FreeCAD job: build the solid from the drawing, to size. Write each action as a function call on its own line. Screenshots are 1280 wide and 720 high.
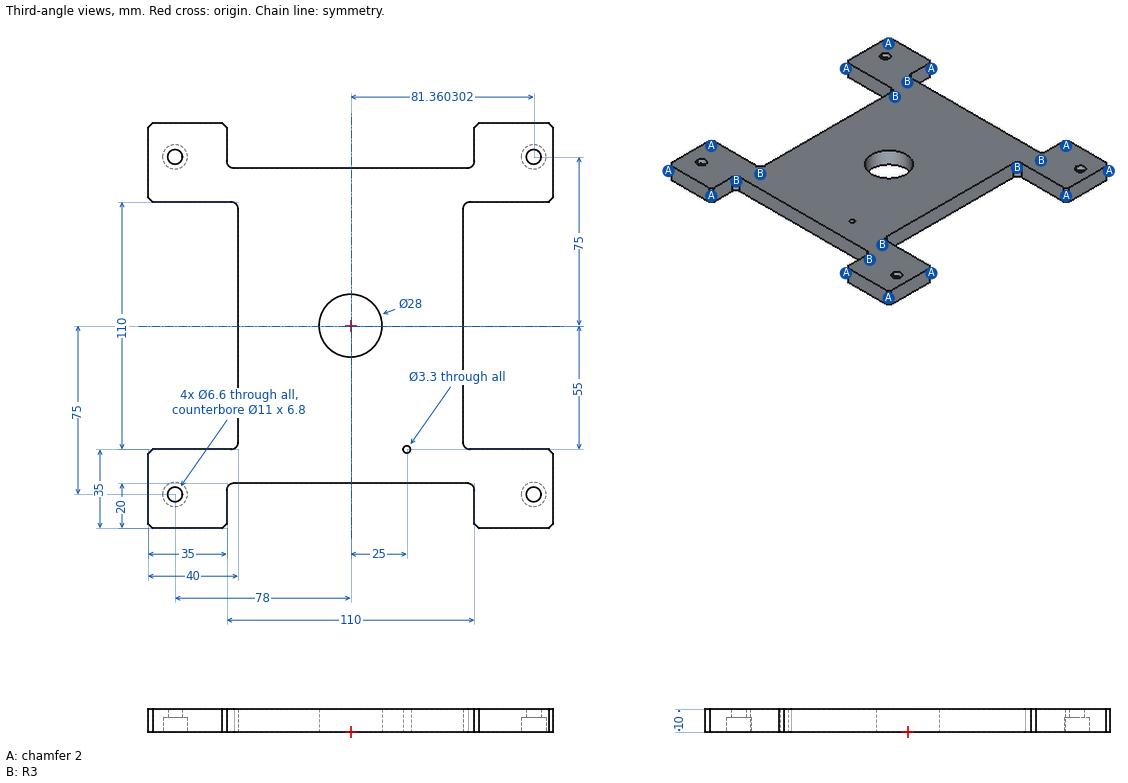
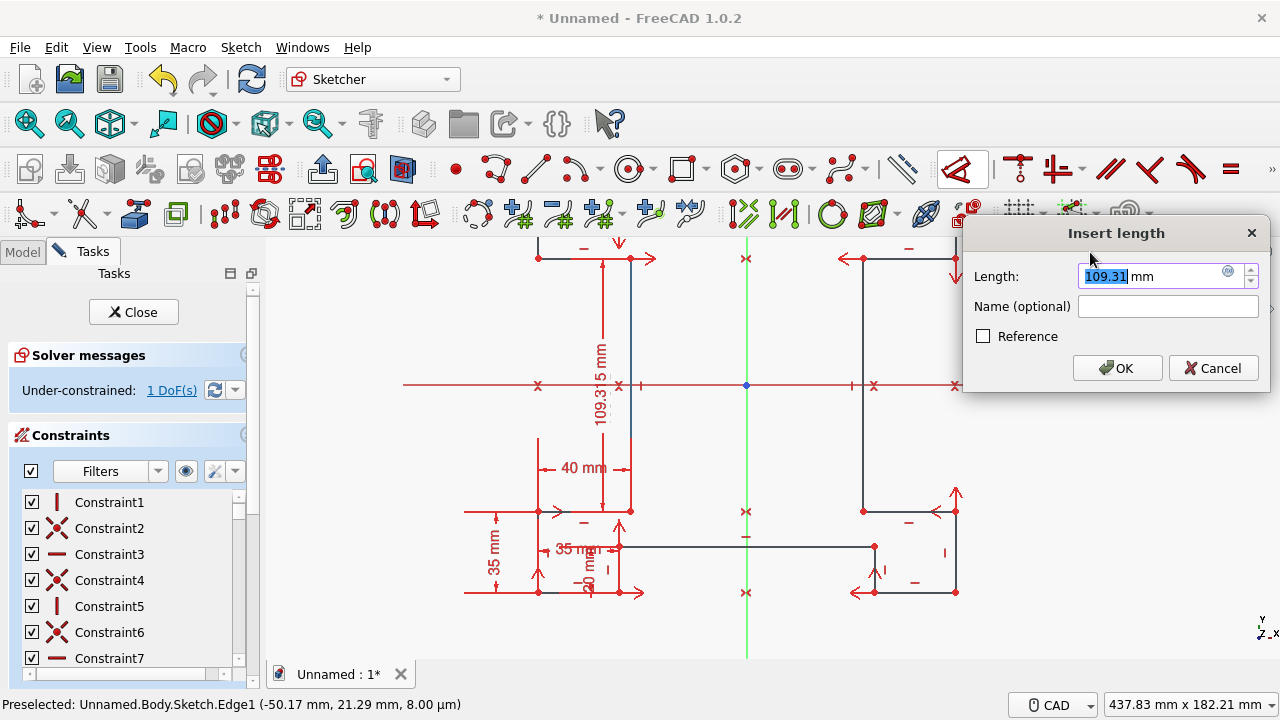
text(110)
key(Return)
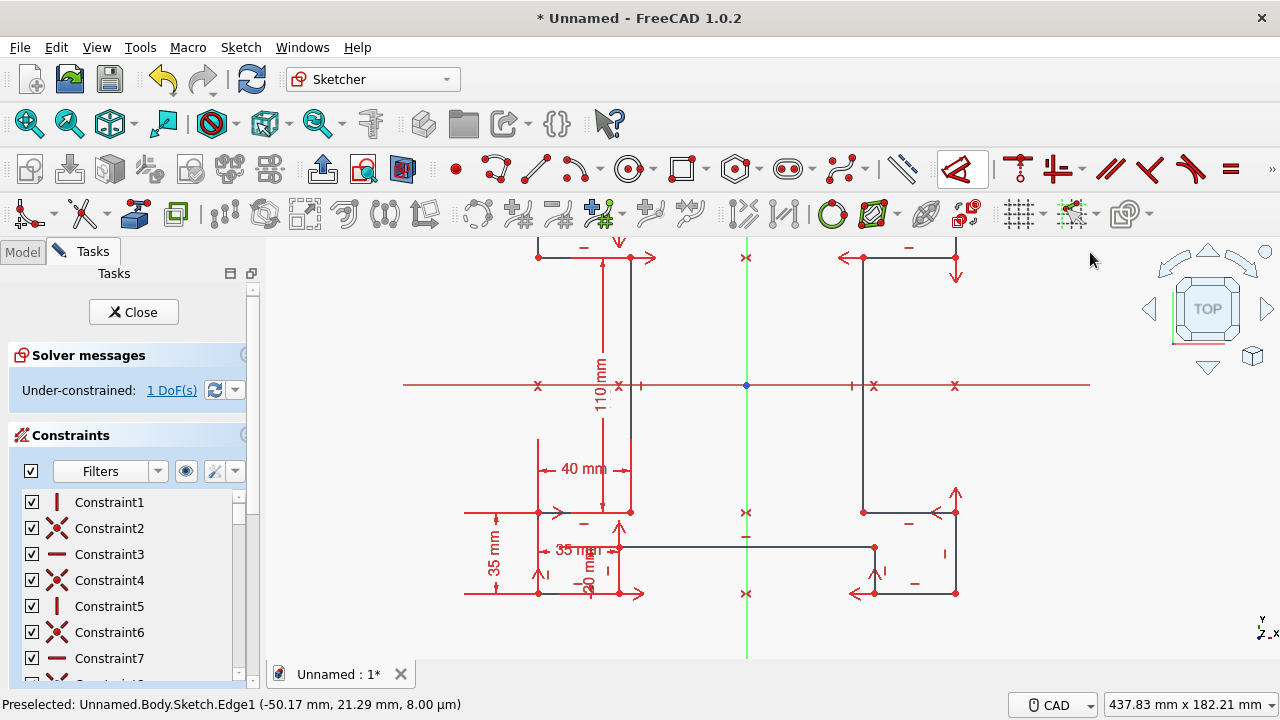
click(696, 547)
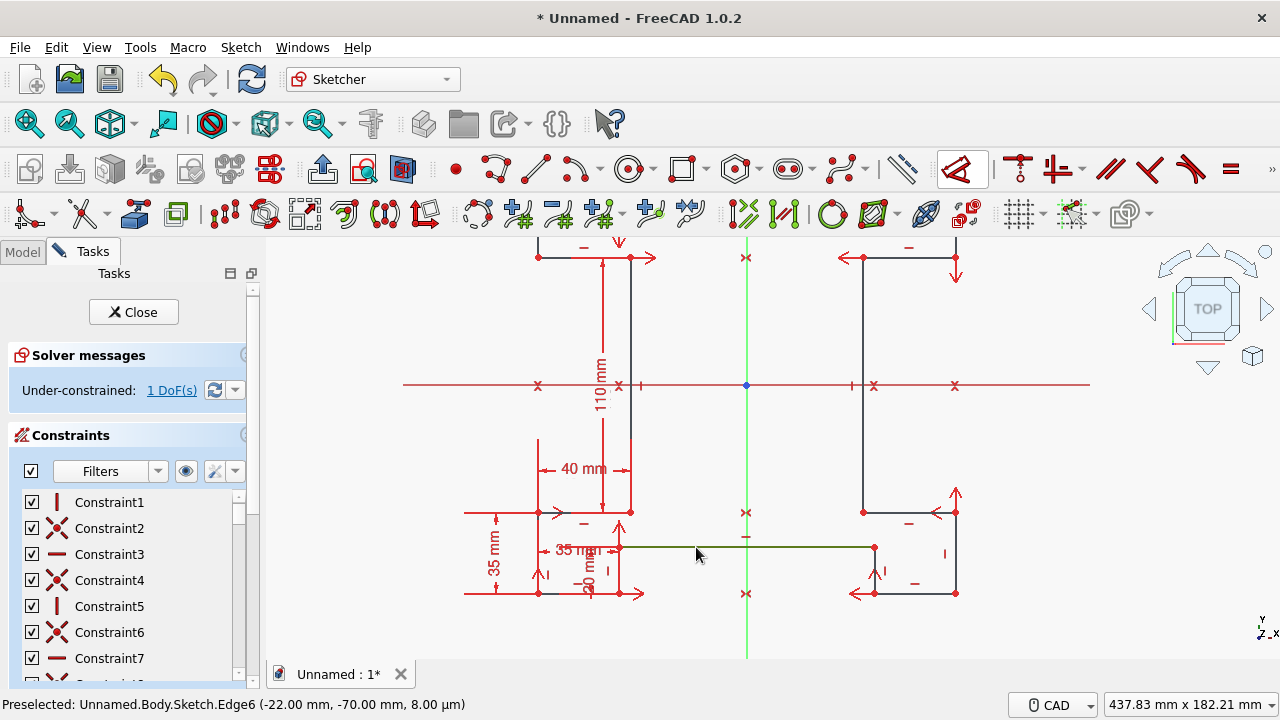
key(l)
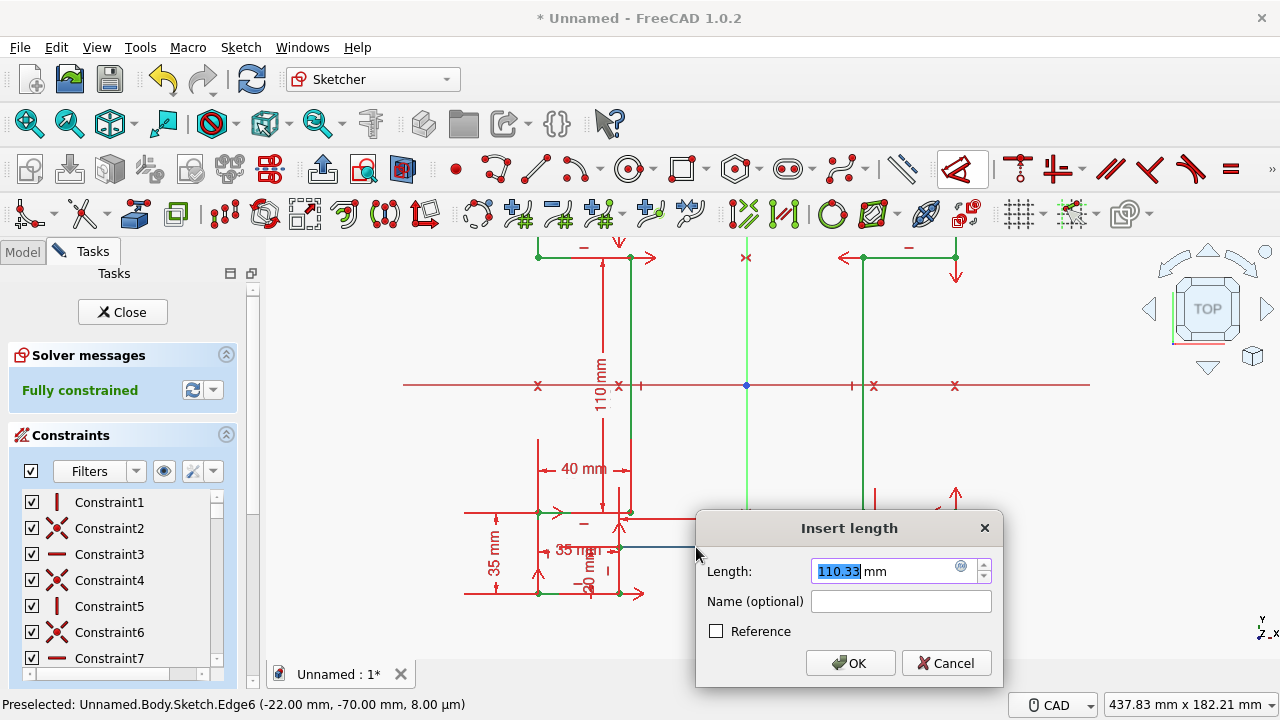
text(110)
key(Return)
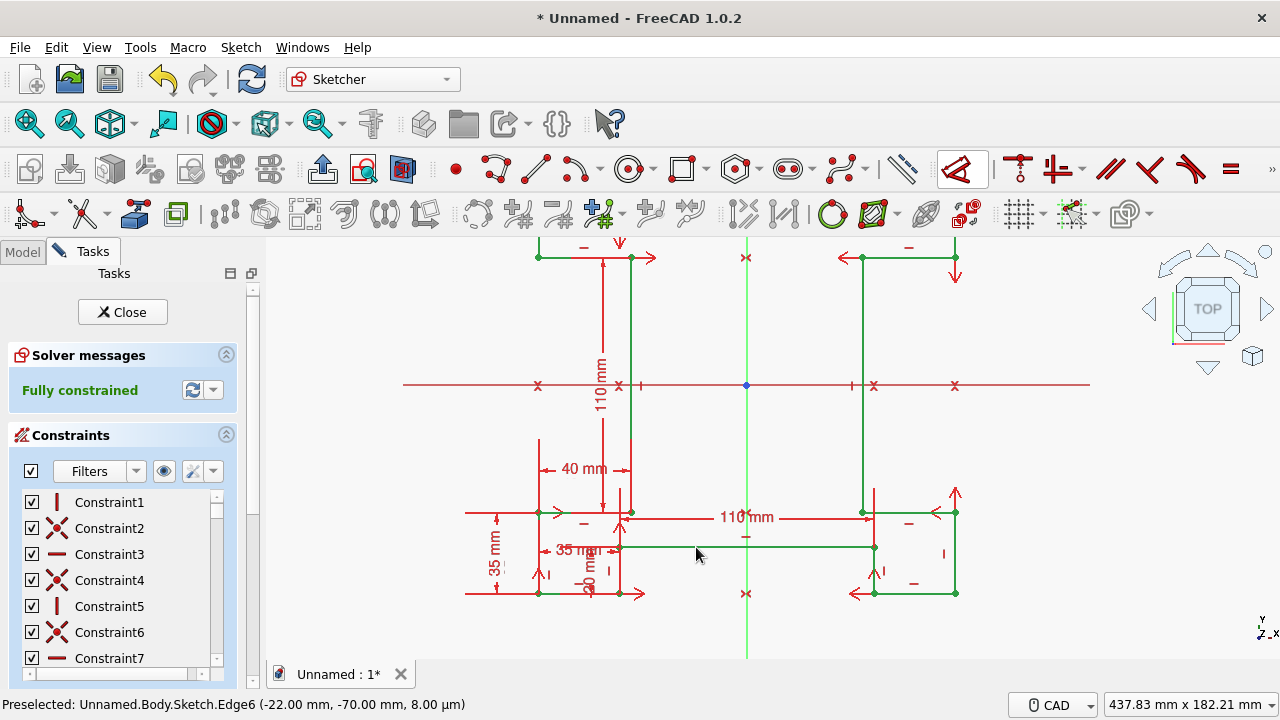
click(123, 312)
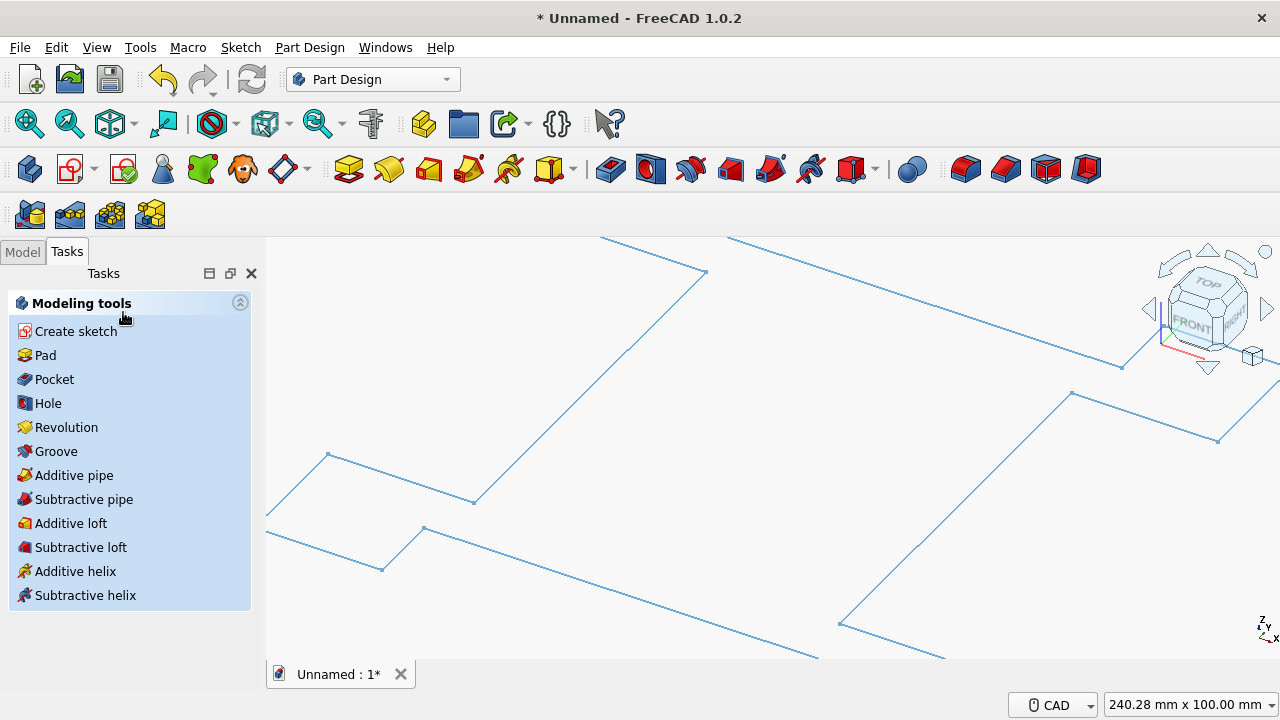
click(350, 170)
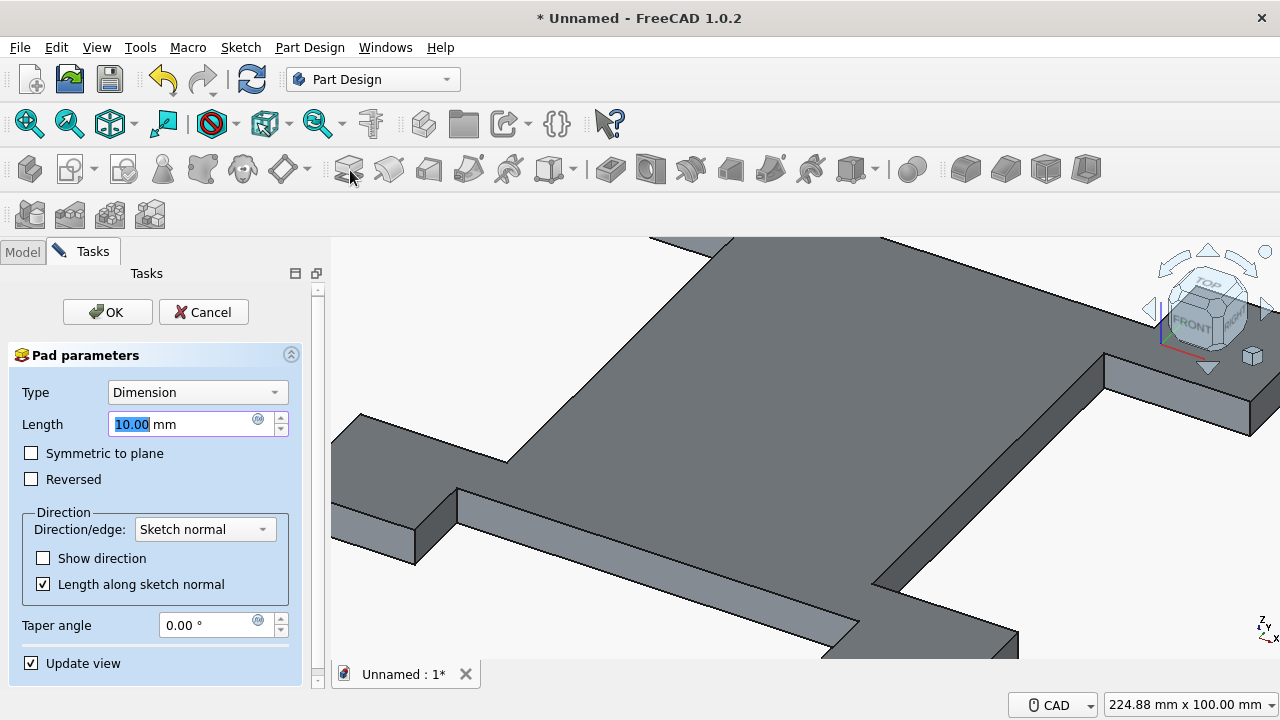
text(10)
key(Tab)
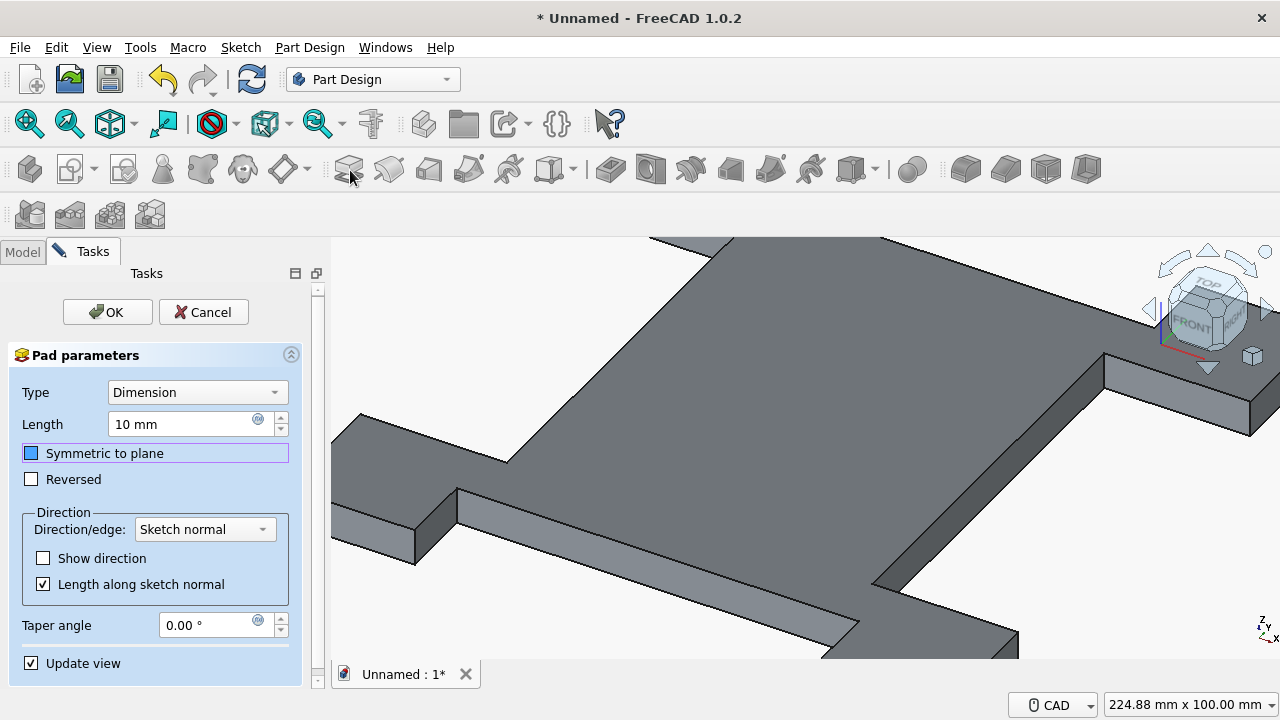
click(108, 312)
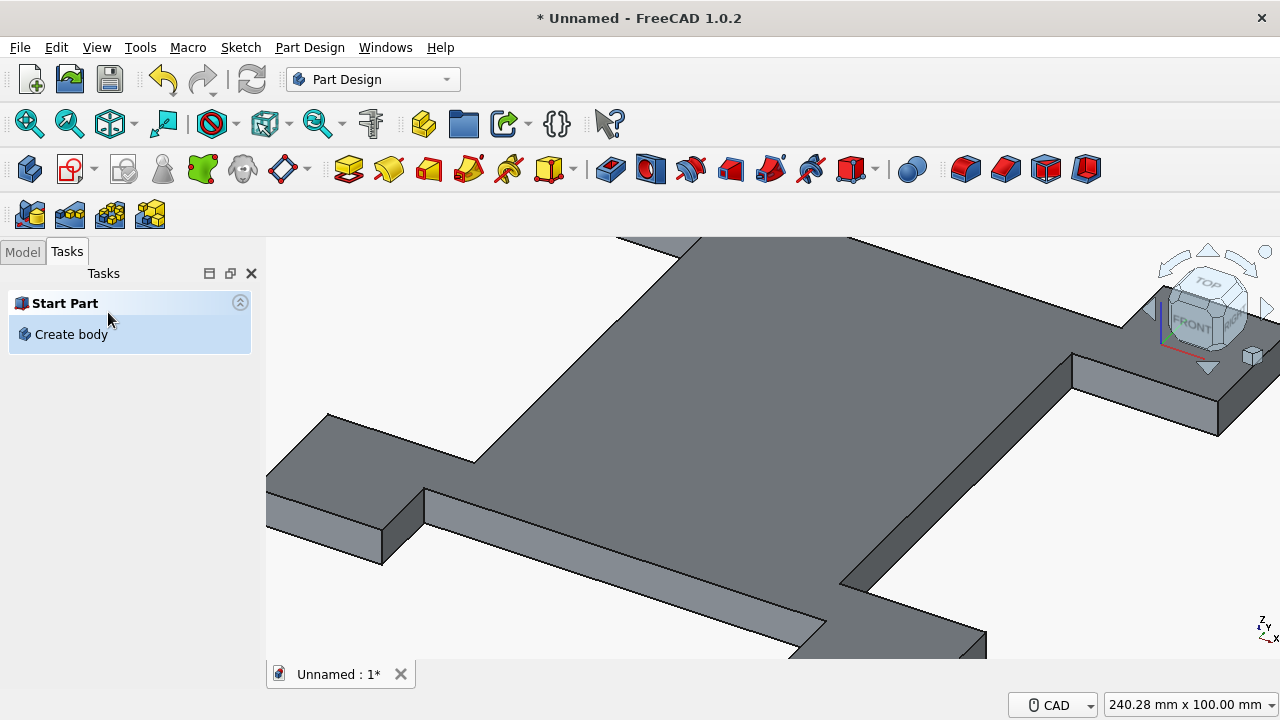
click(30, 124)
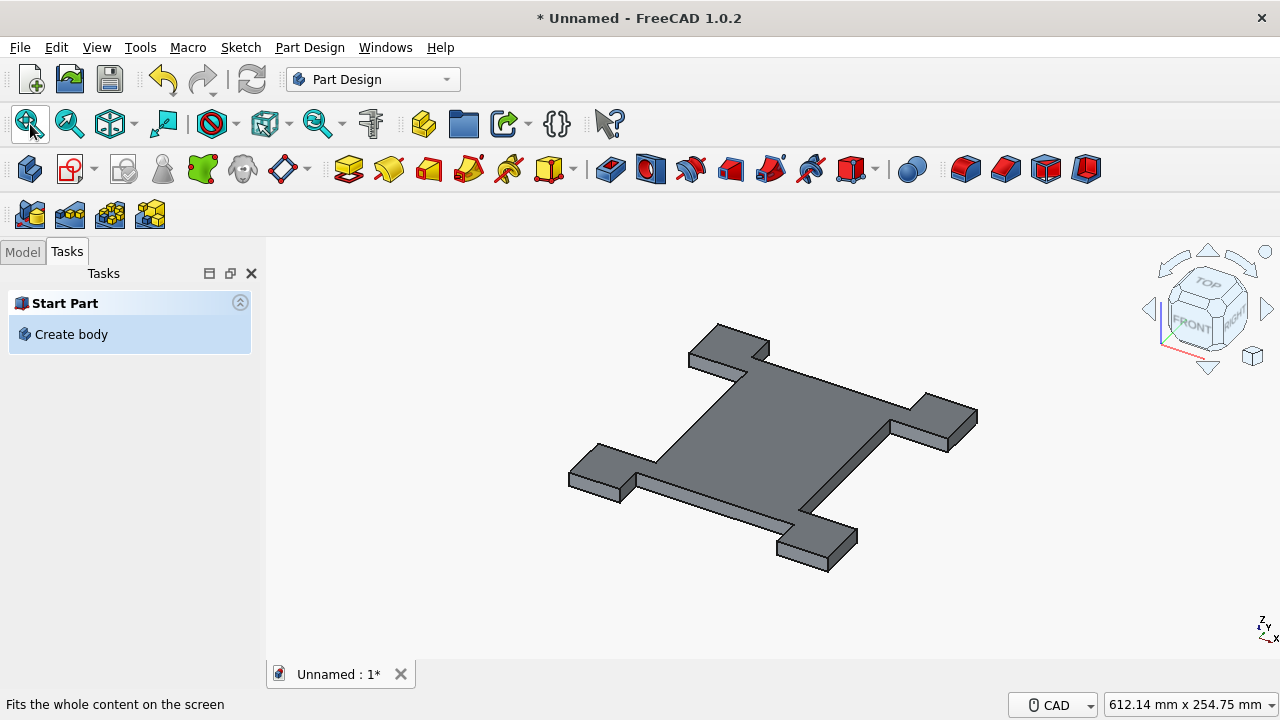
key(5)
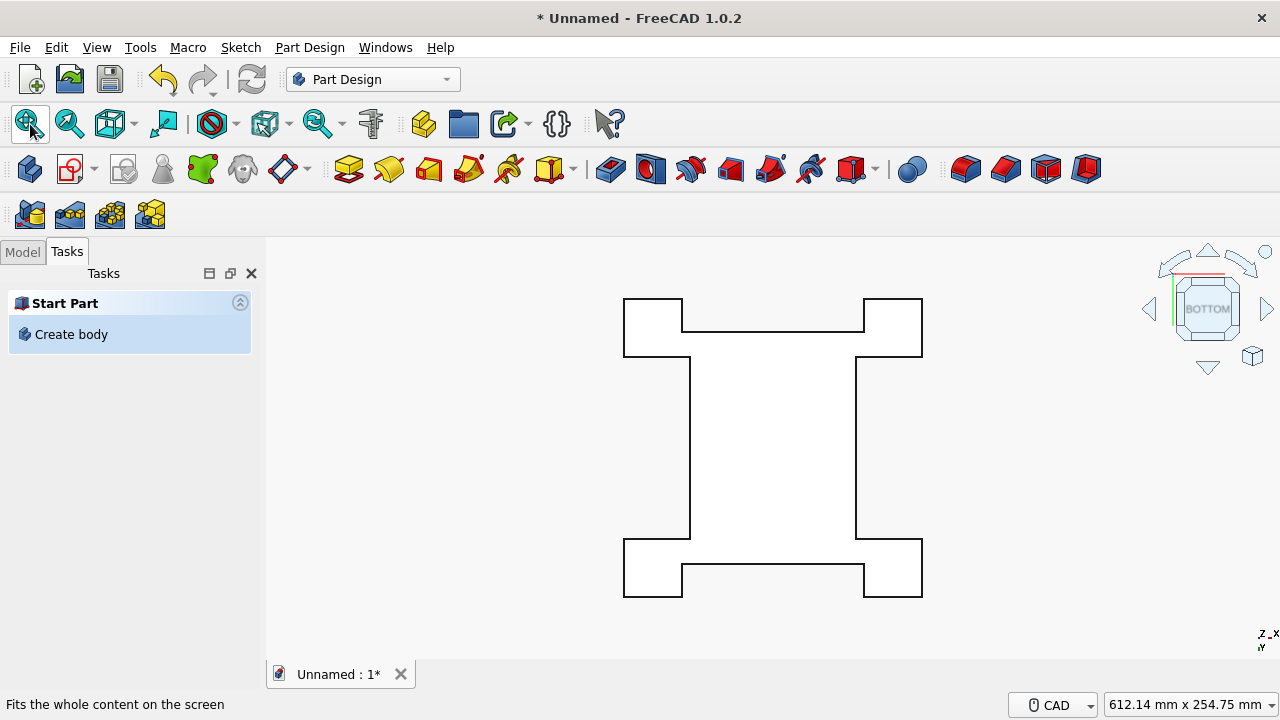
click(773, 447)